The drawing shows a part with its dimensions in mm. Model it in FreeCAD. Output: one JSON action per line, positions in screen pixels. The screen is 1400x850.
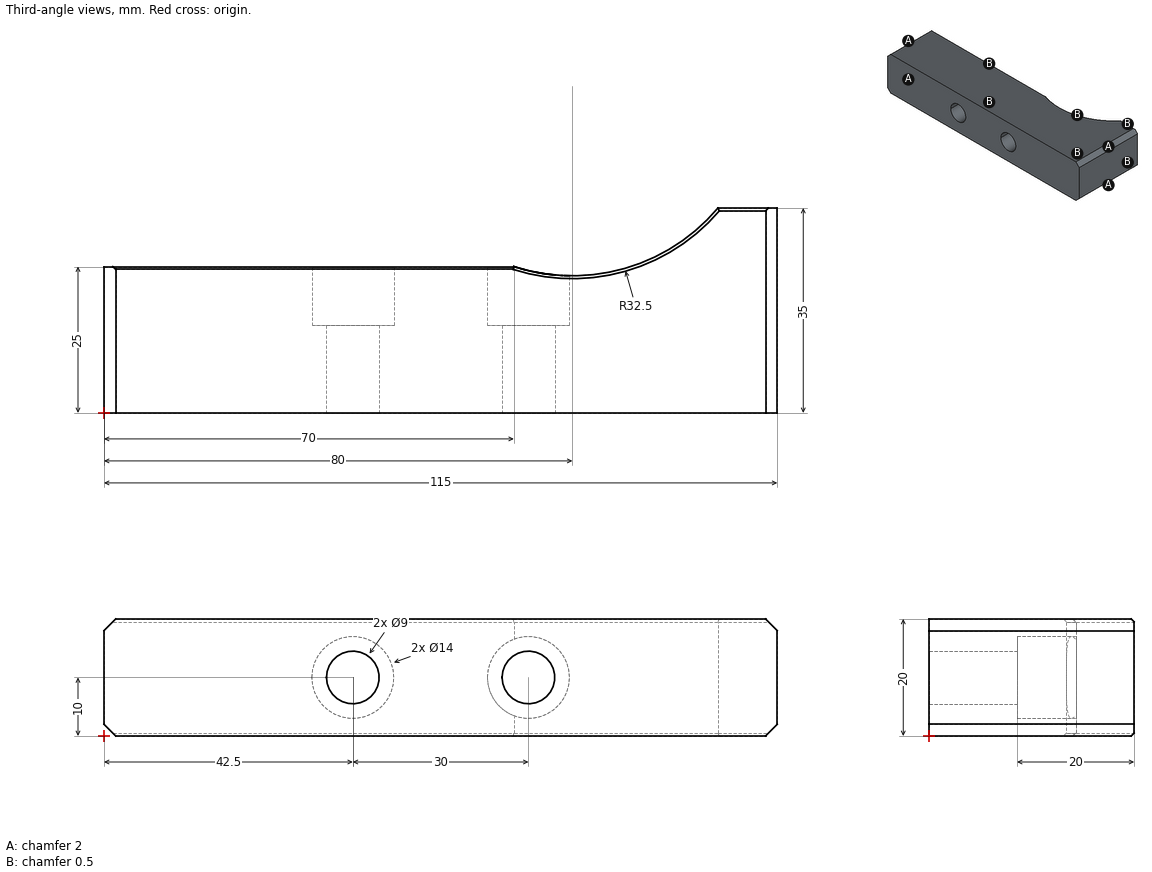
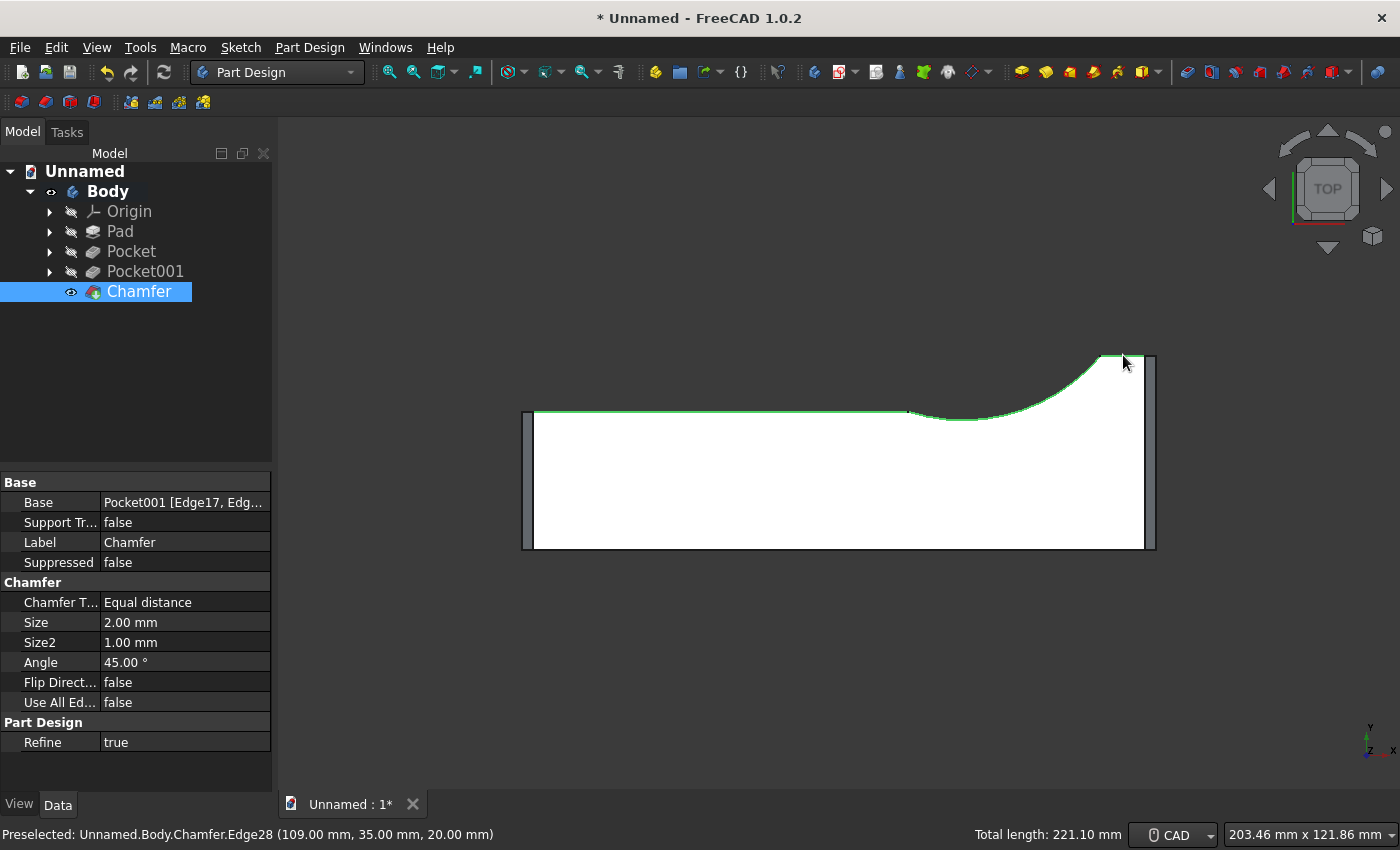
{"action": "key", "text": "1"}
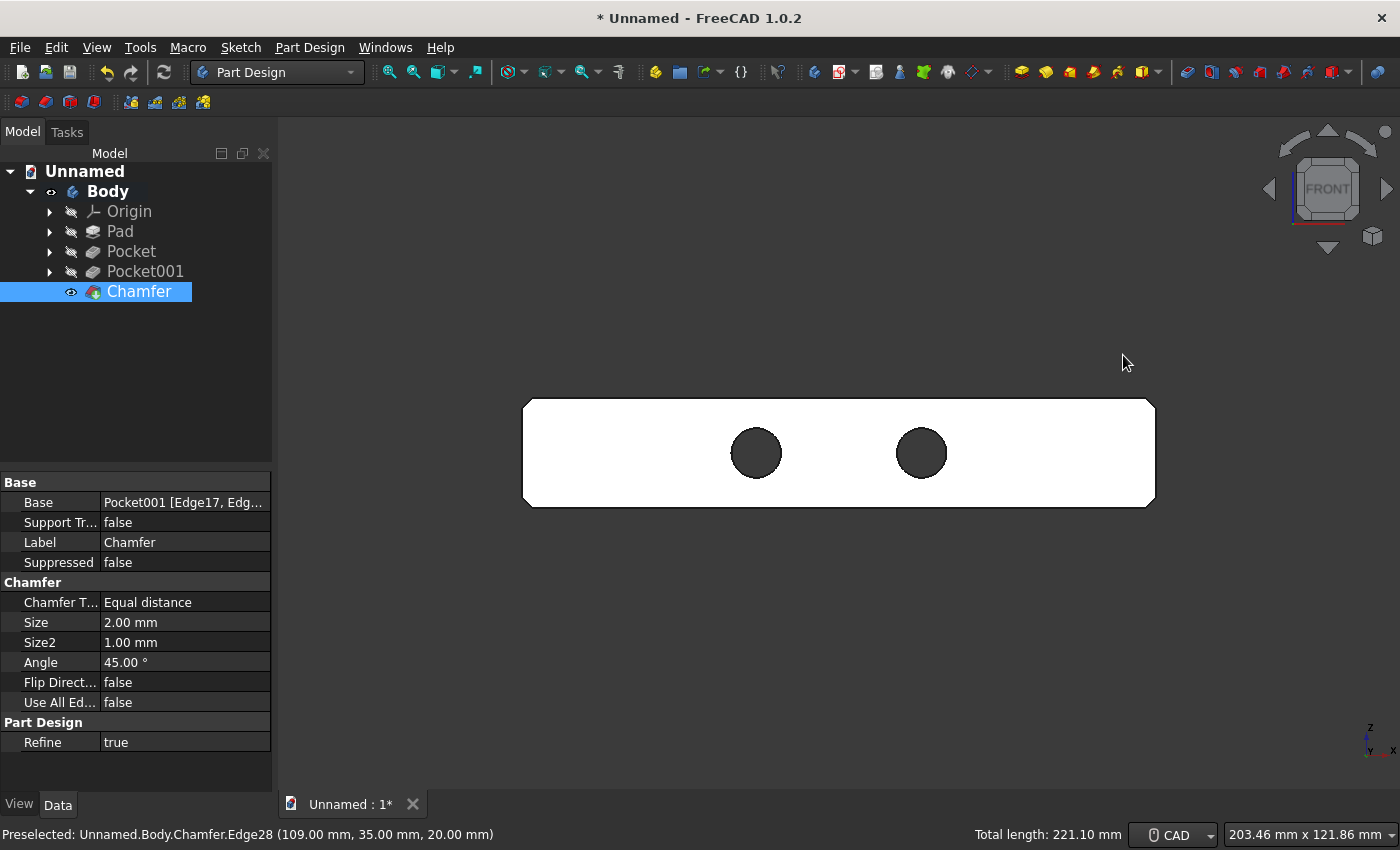
{"action": "key", "text": "3"}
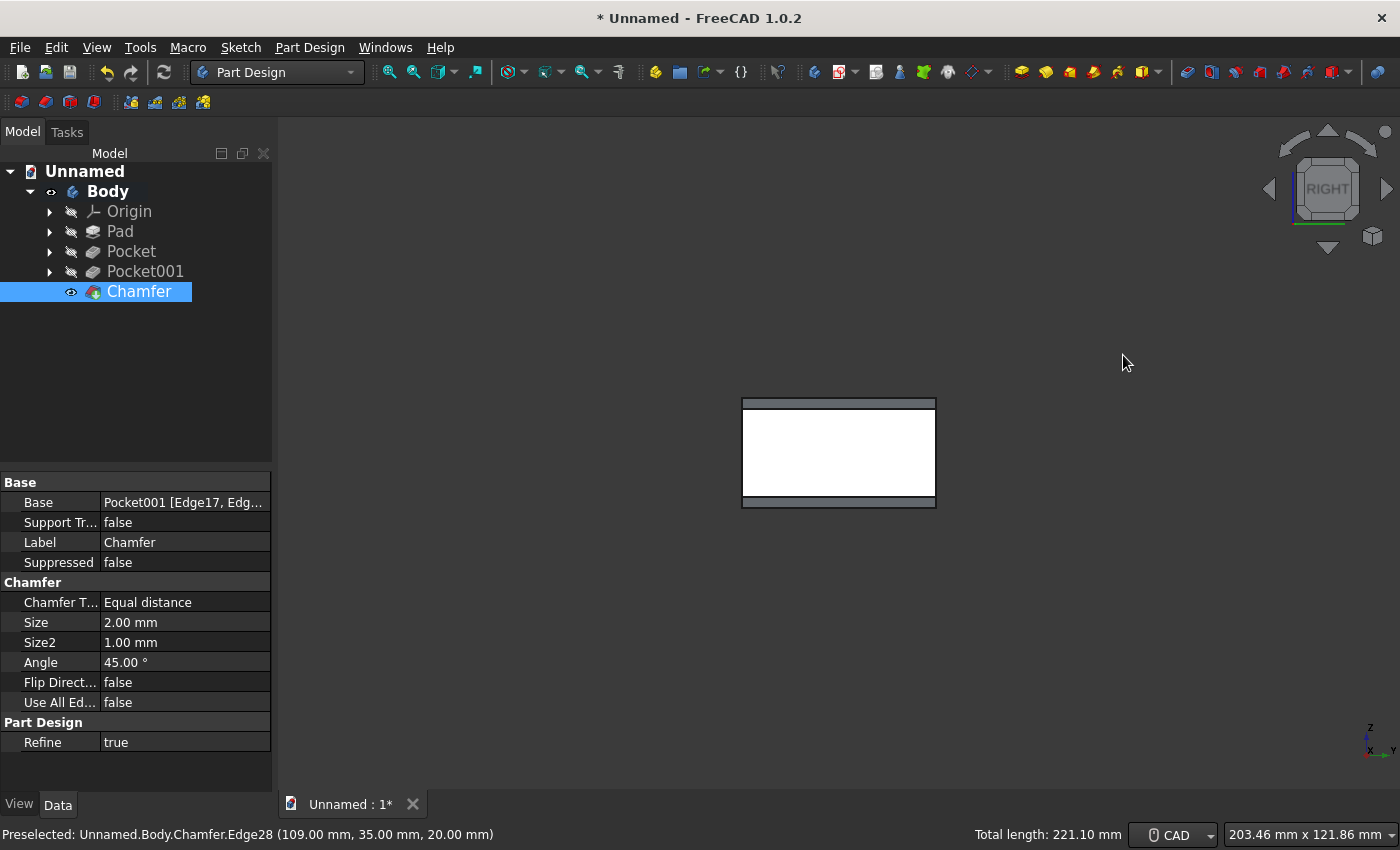
{"action": "left_click", "coordinate": [390, 72]}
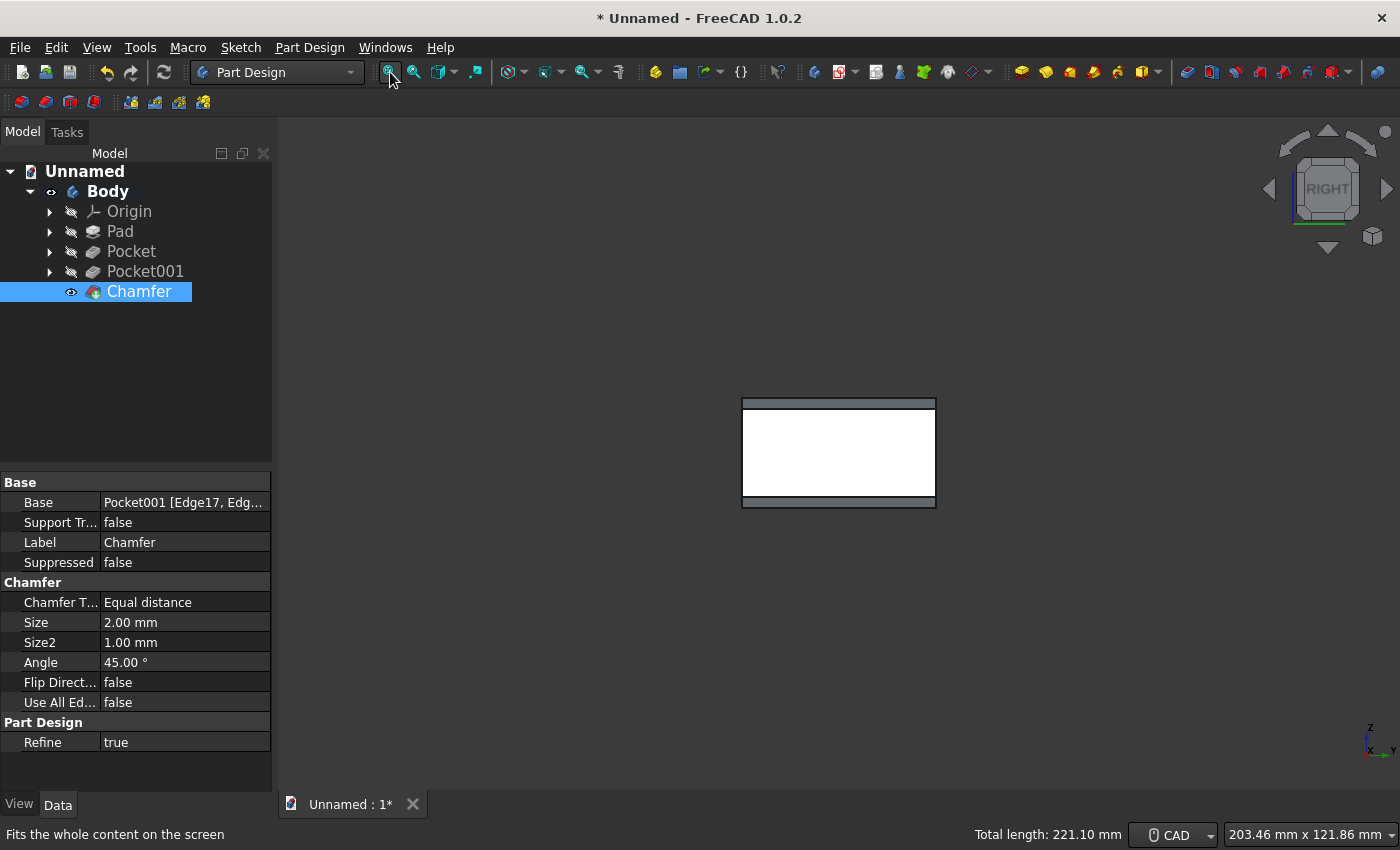
{"action": "key", "text": "5"}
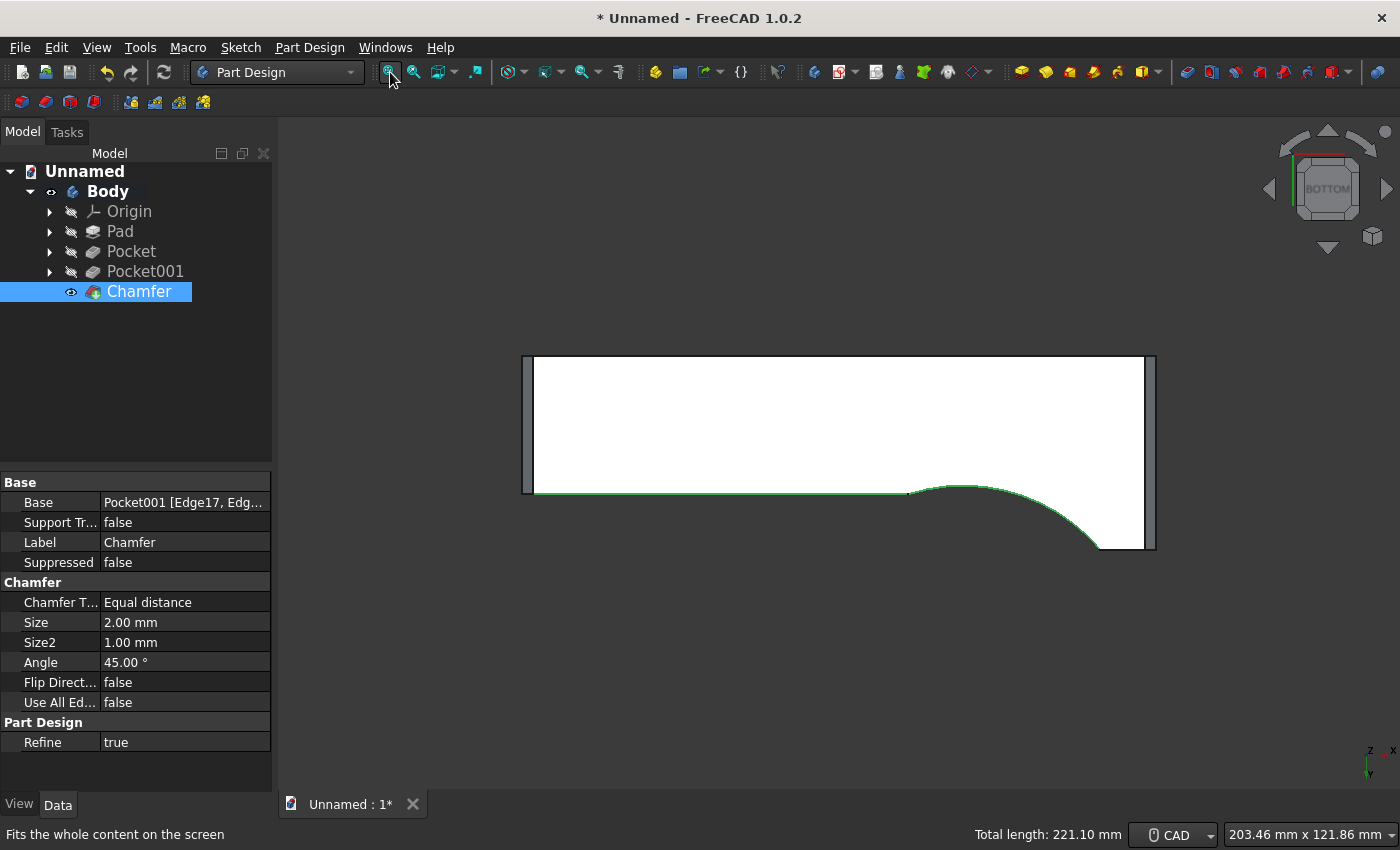
{"action": "key", "text": "4"}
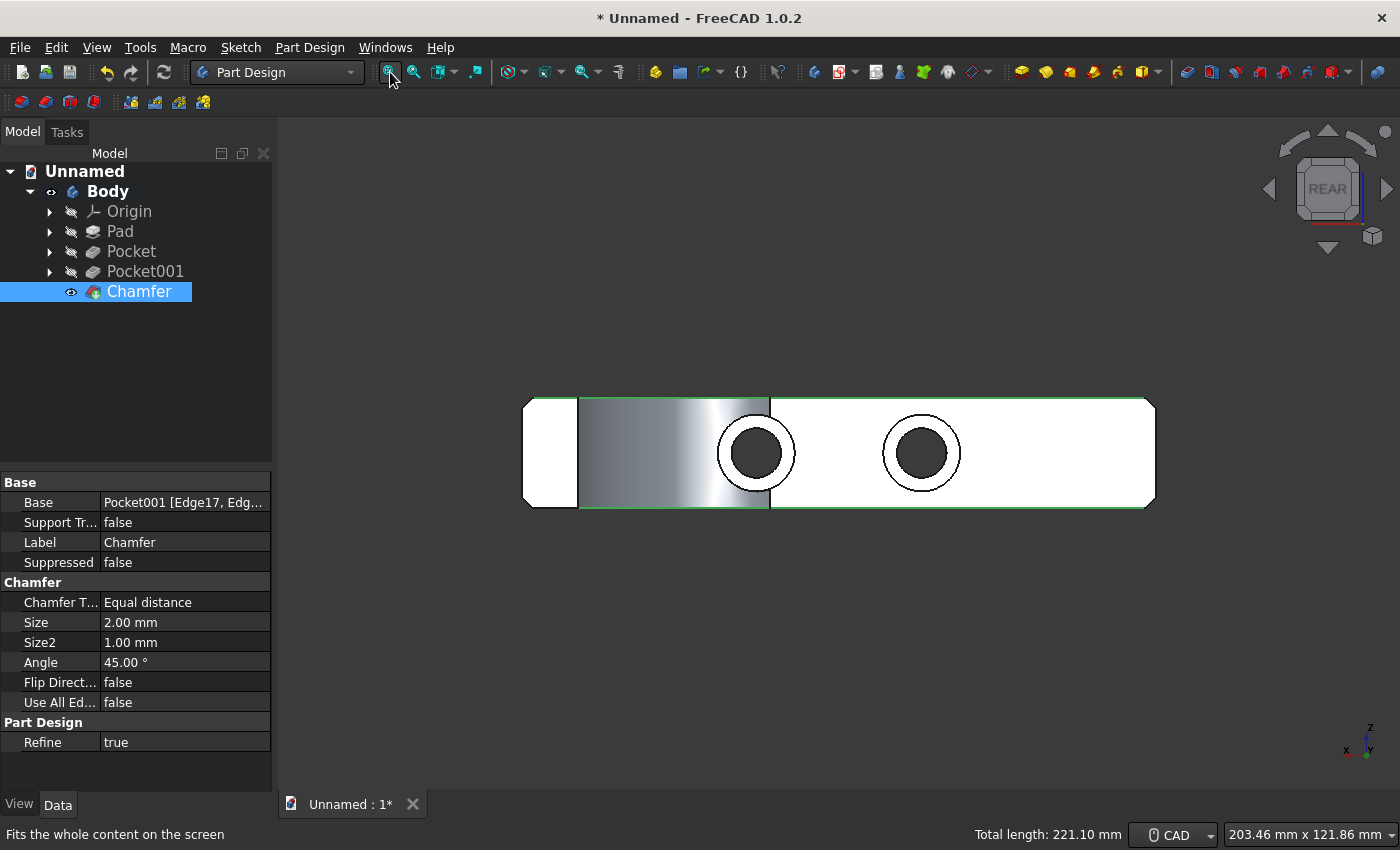
{"action": "left_click", "coordinate": [555, 507], "text": "ctrl"}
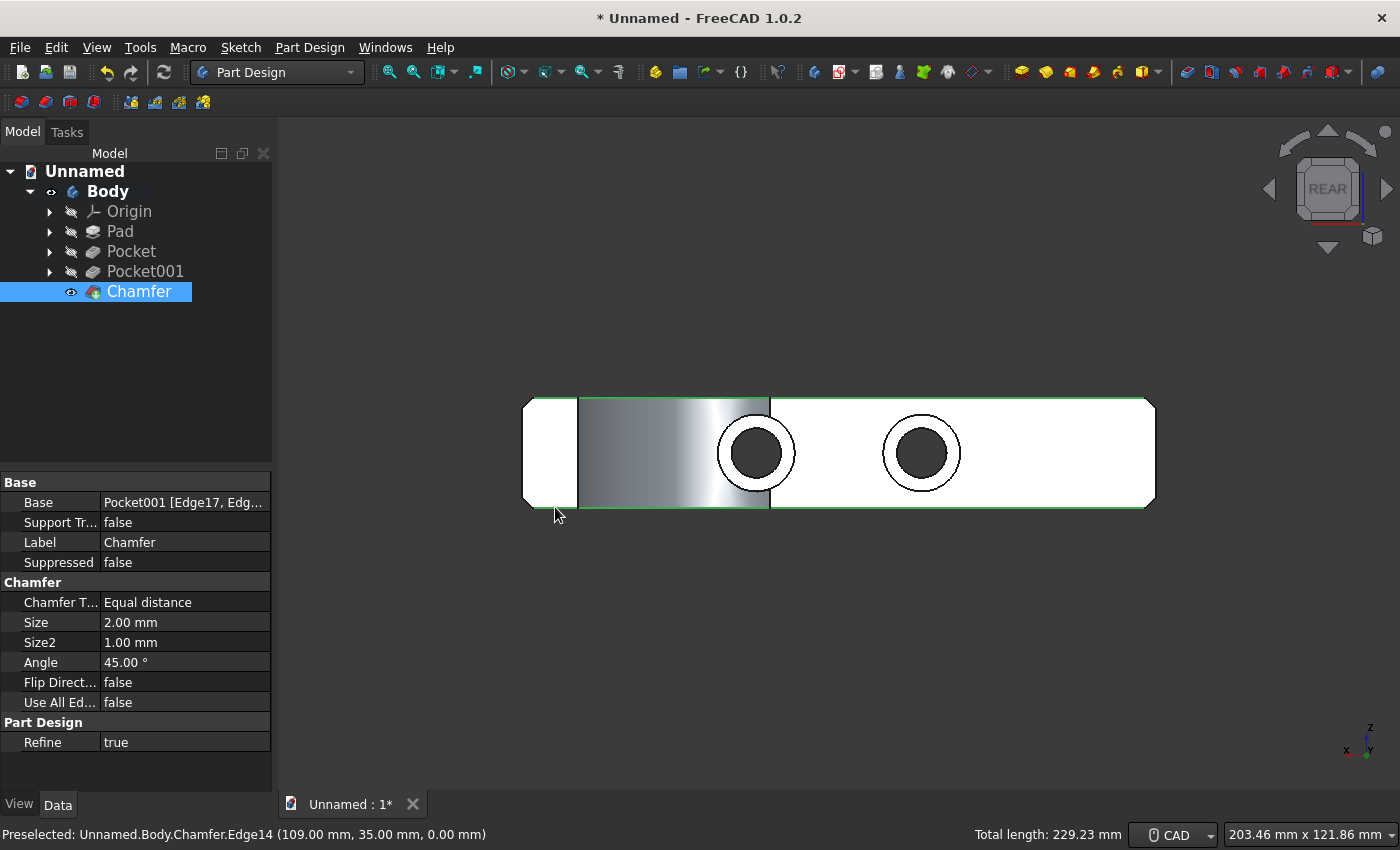
{"action": "left_click", "coordinate": [46, 102]}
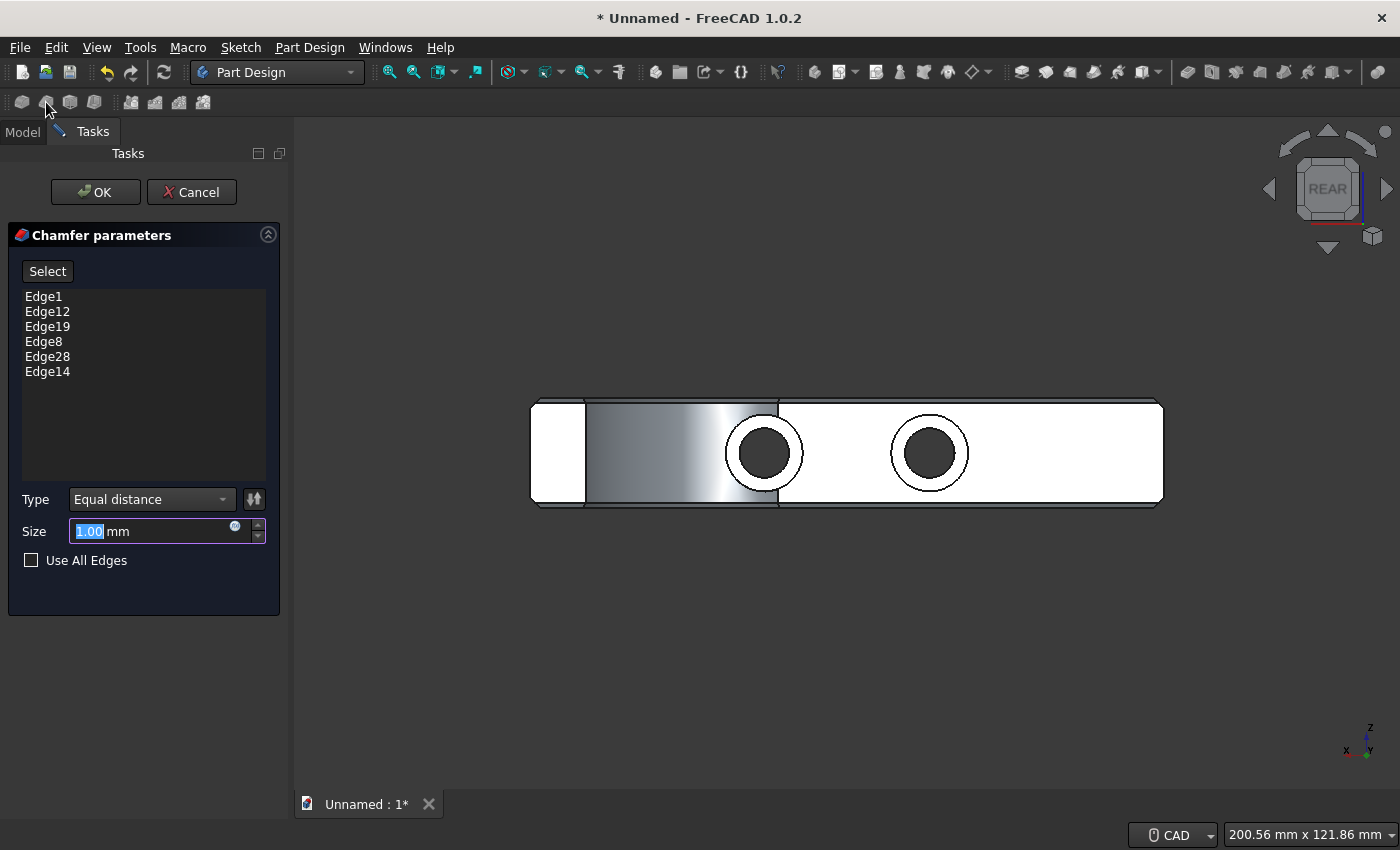
{"action": "type", "text": "0.5"}
{"action": "key", "text": "Tab"}